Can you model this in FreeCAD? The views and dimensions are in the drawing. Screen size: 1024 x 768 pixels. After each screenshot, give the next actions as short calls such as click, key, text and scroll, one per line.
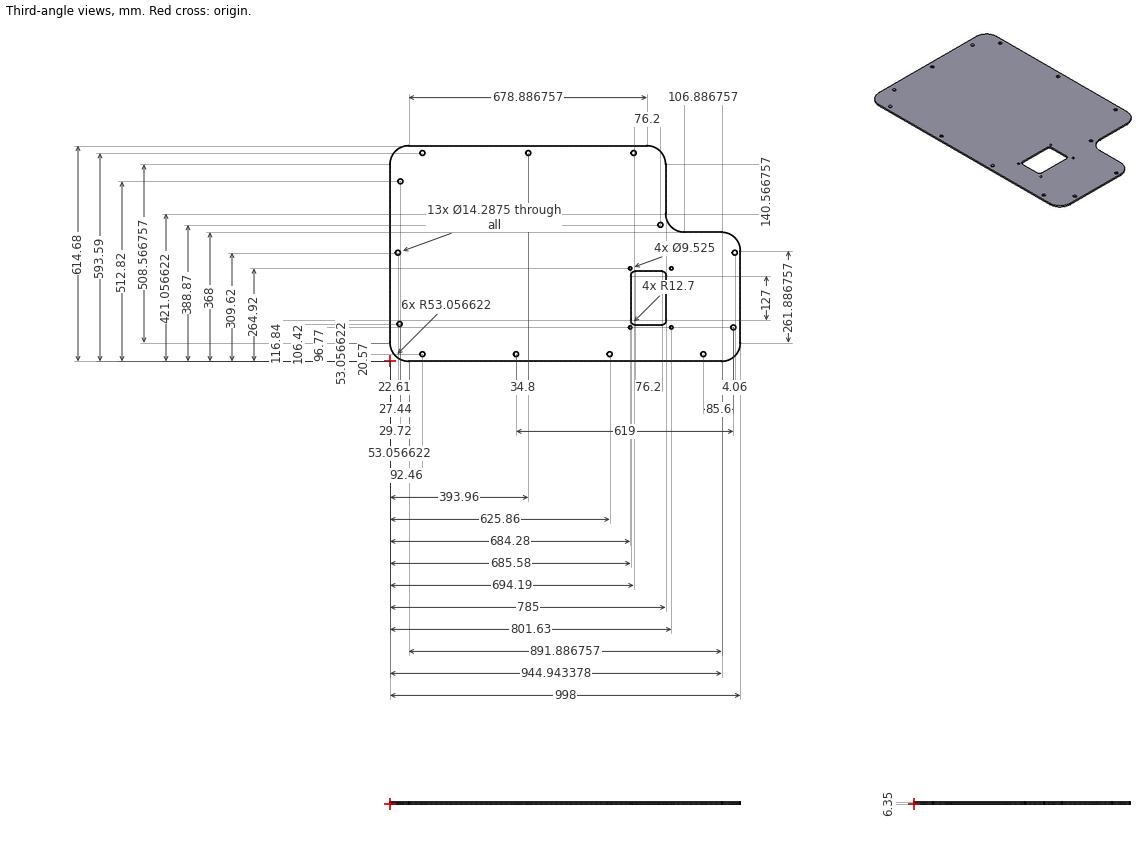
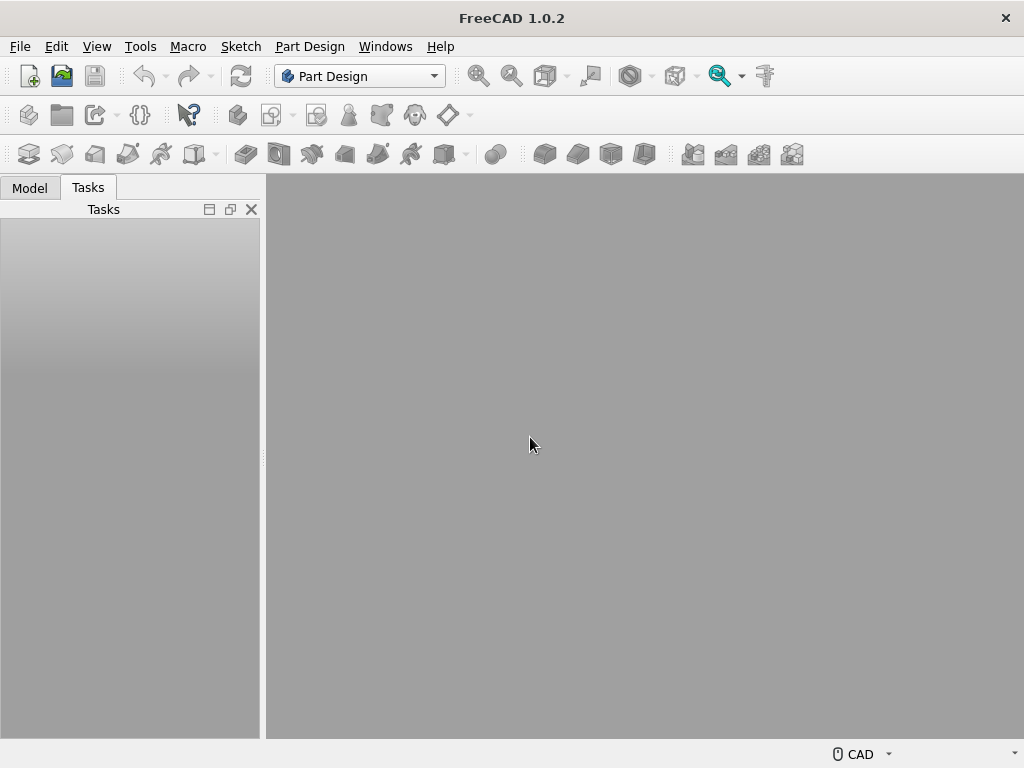
click(29, 76)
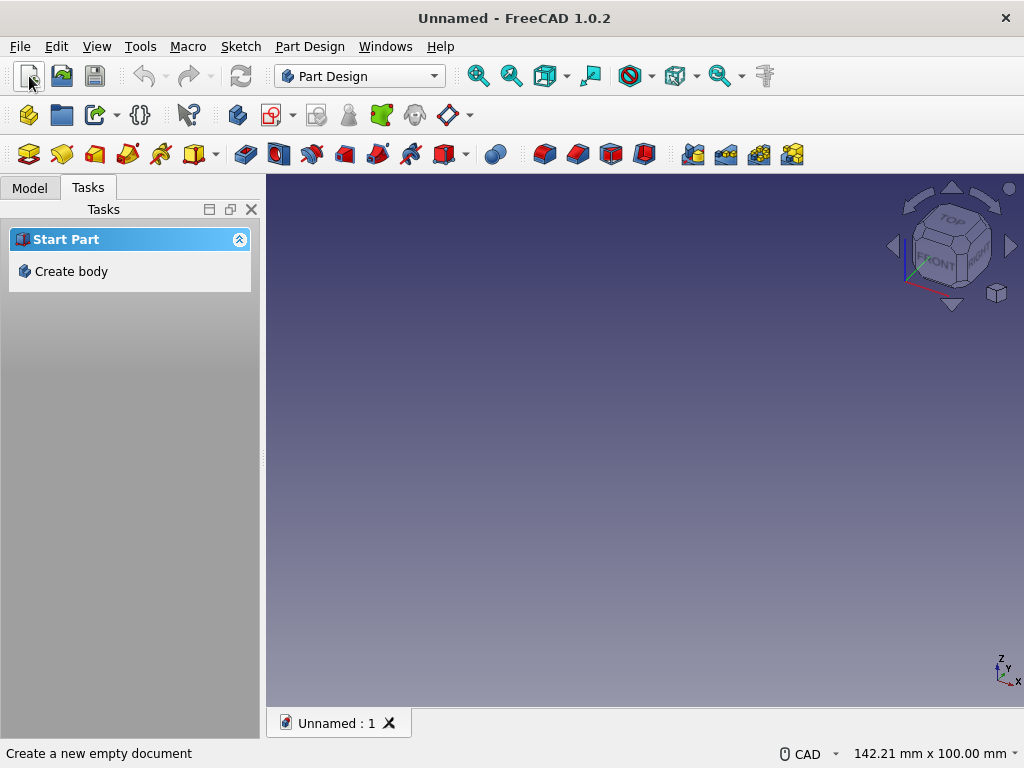
click(270, 116)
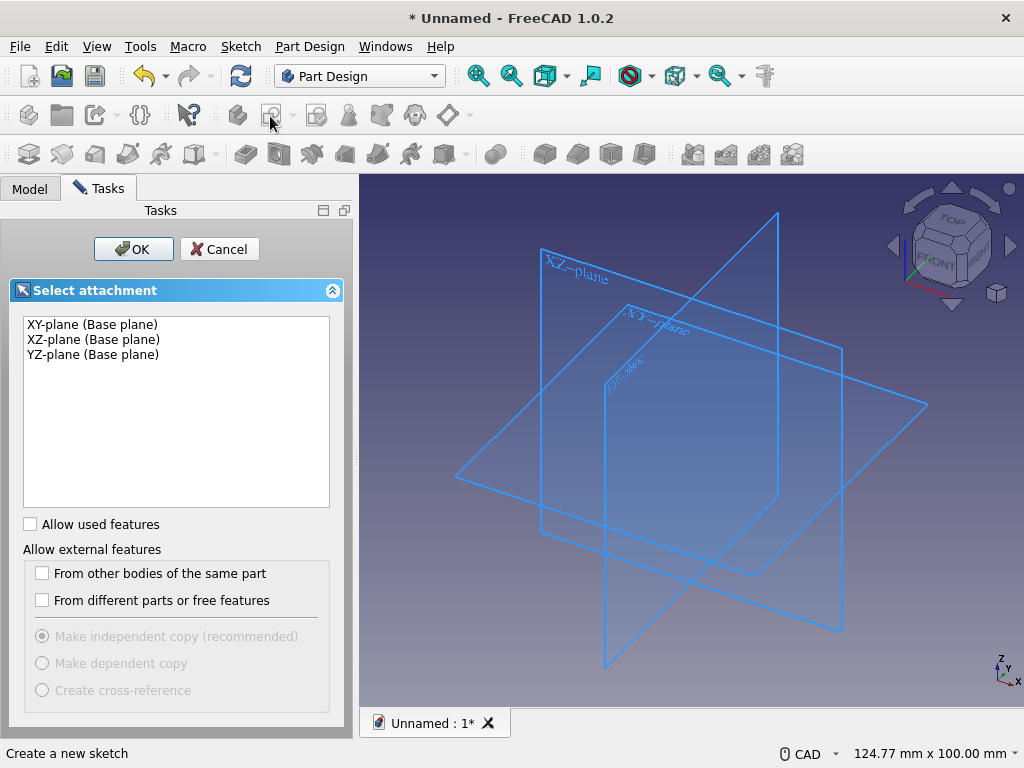
click(84, 324)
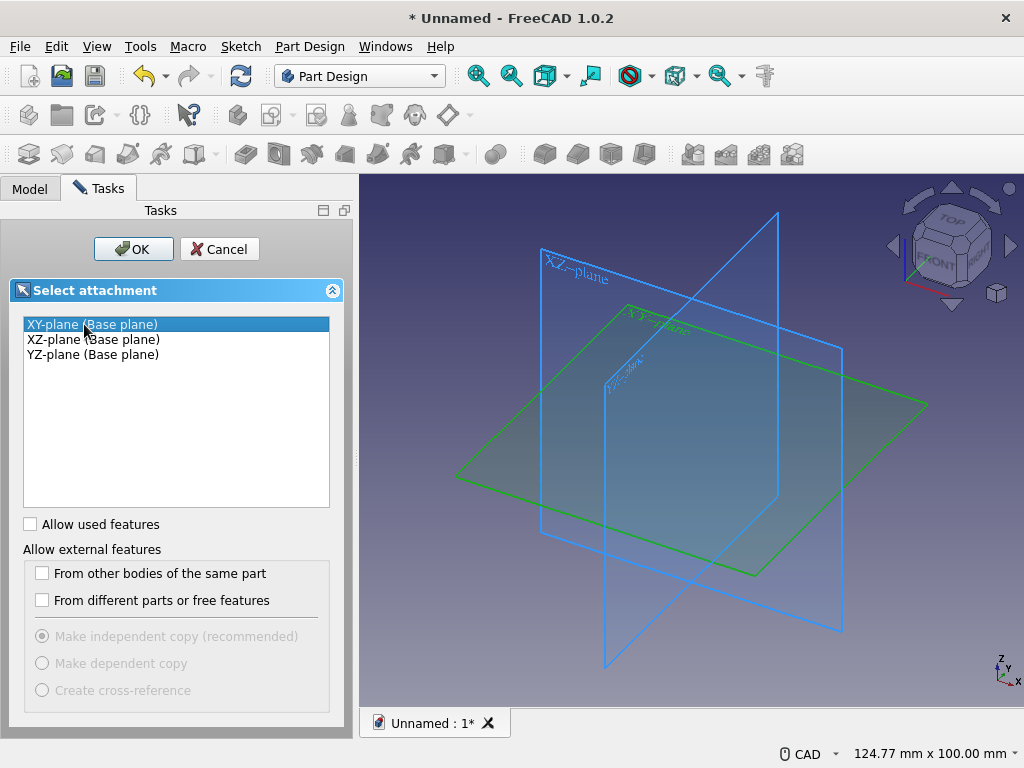
click(134, 249)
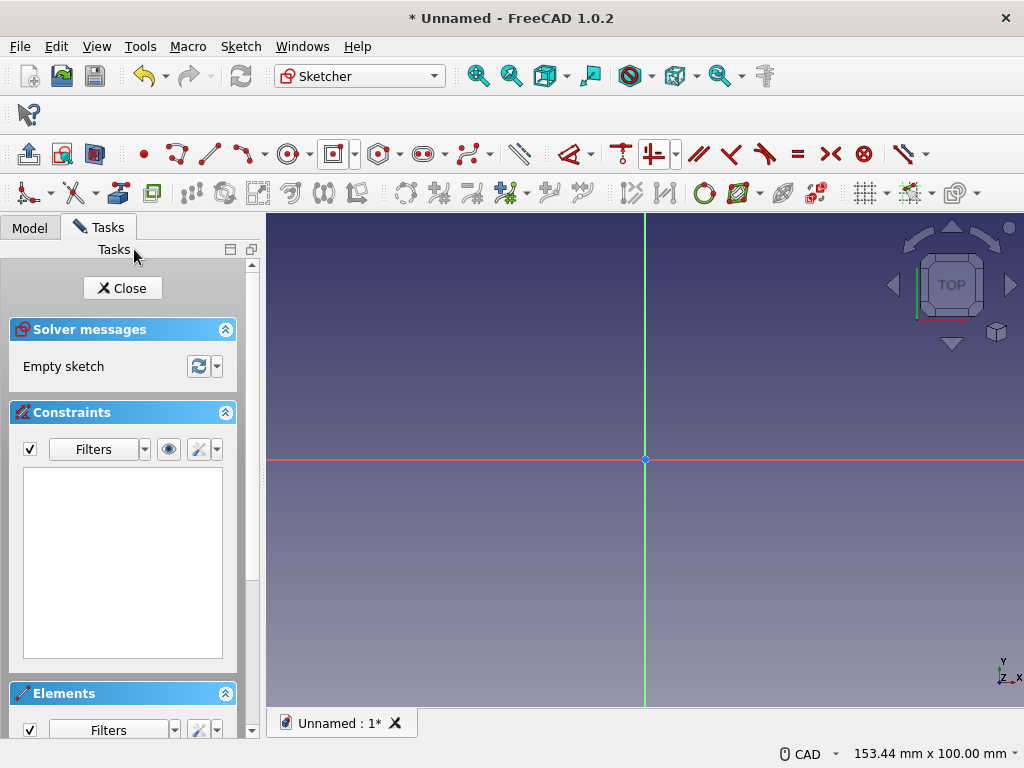
scroll(373, 582, down, 13)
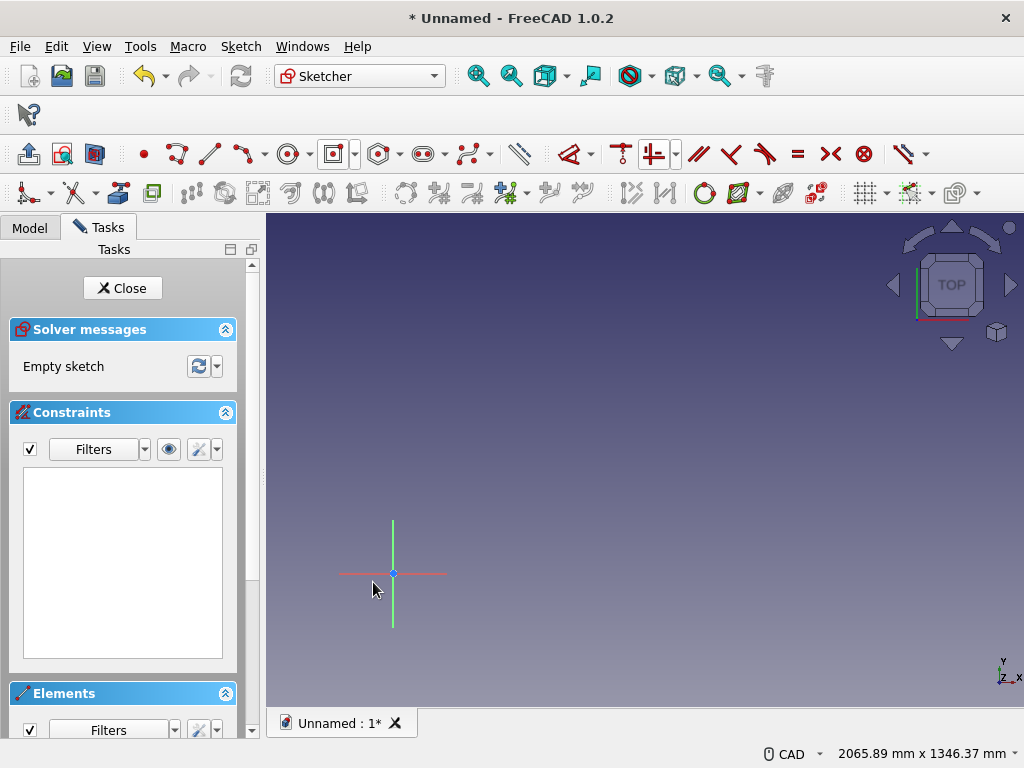
click(210, 154)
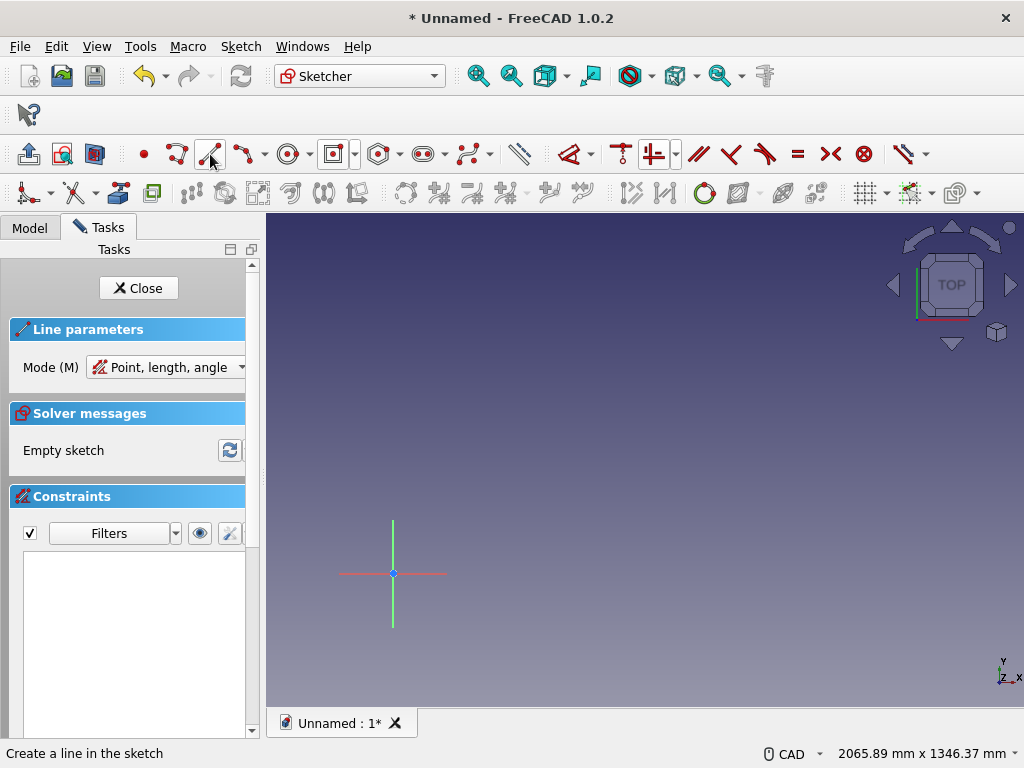
click(393, 368)
click(402, 554)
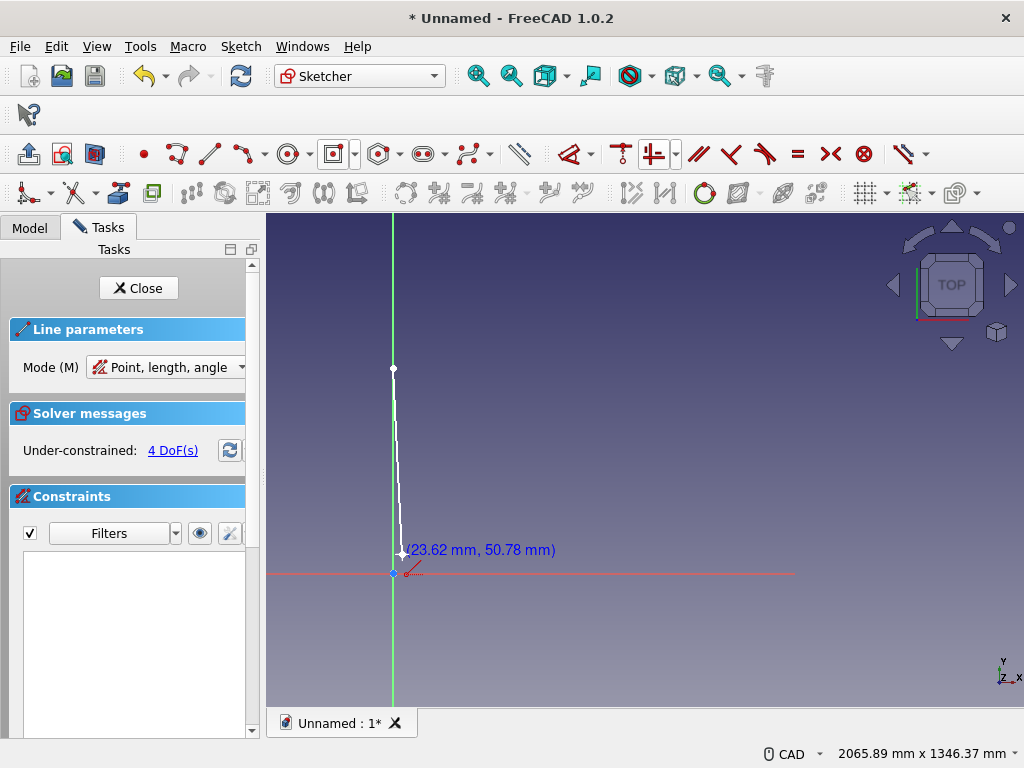
click(413, 574)
click(740, 565)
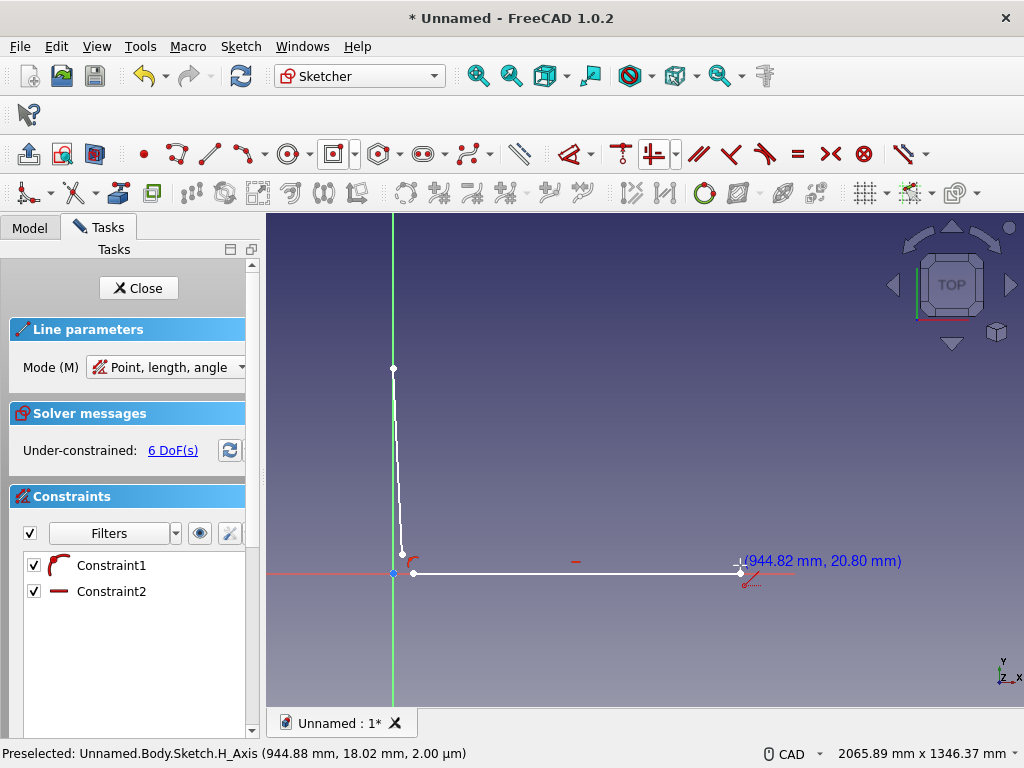
click(760, 554)
click(760, 458)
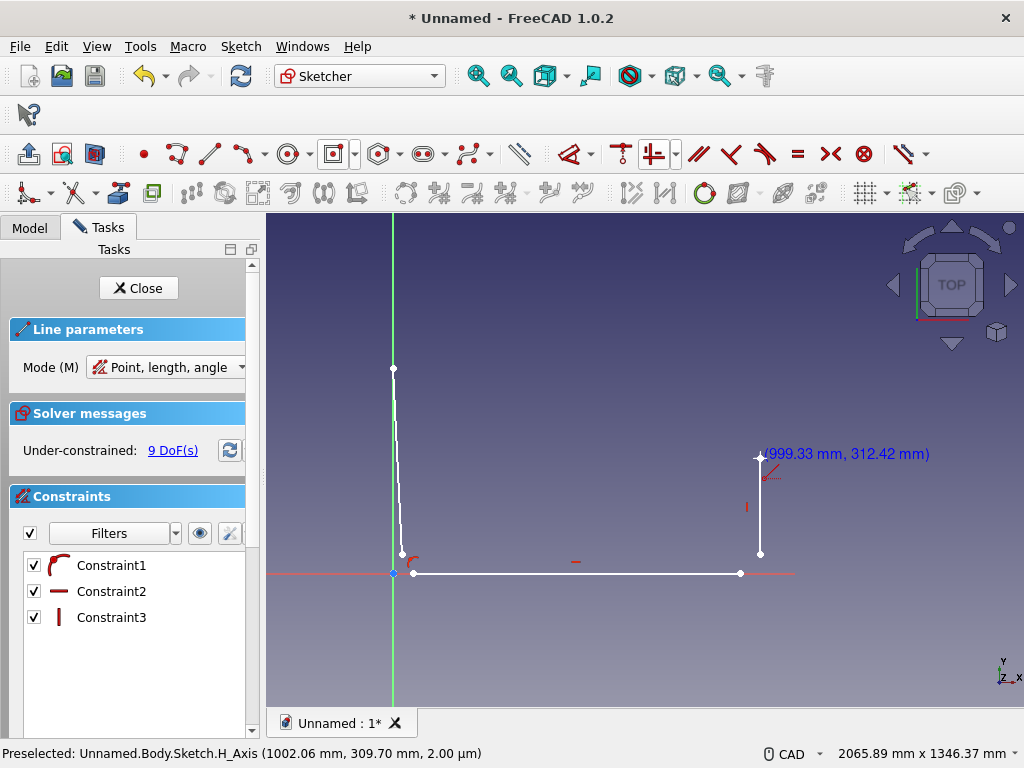
click(740, 439)
click(701, 439)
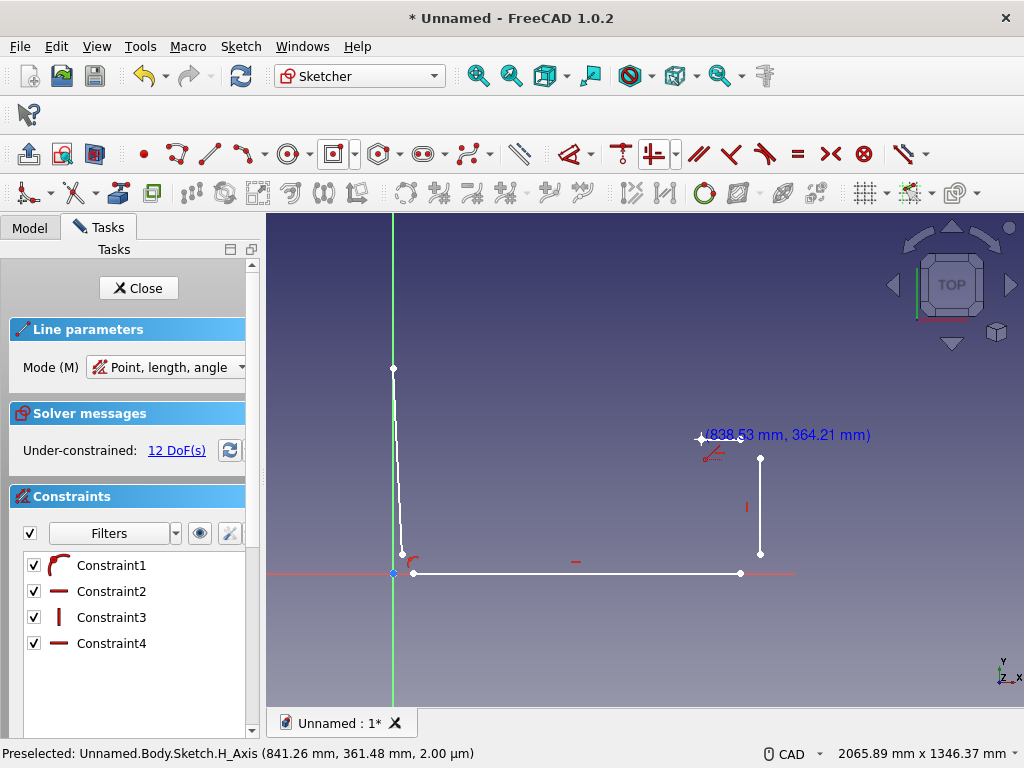
click(681, 419)
click(681, 368)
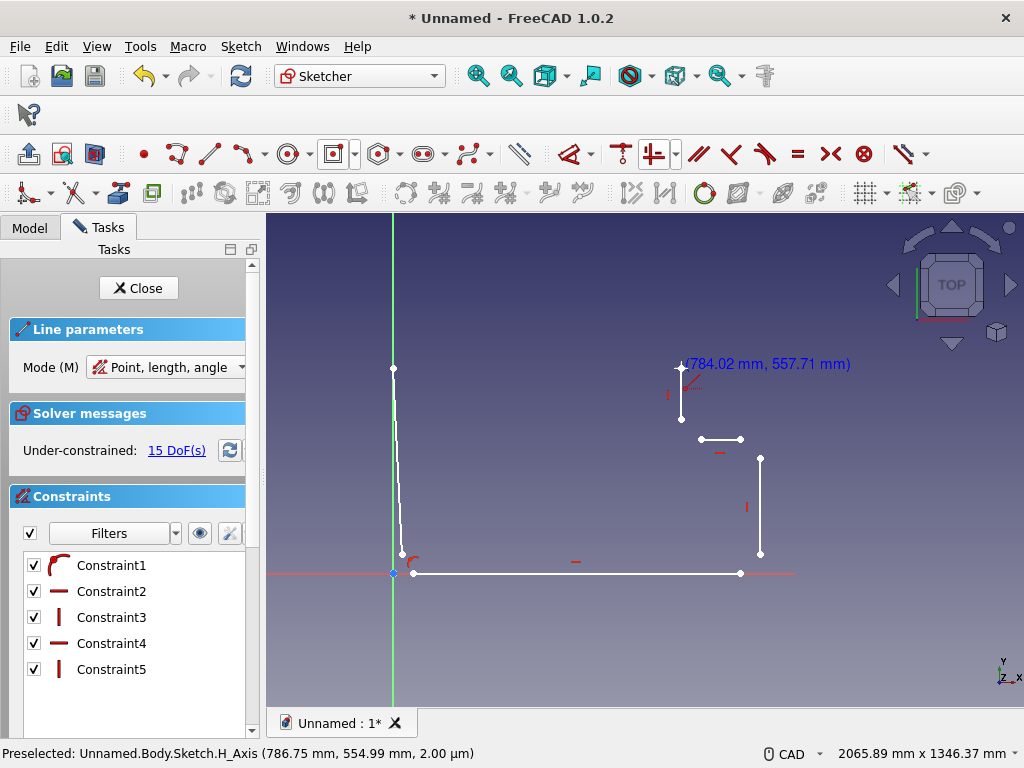
click(662, 348)
click(413, 348)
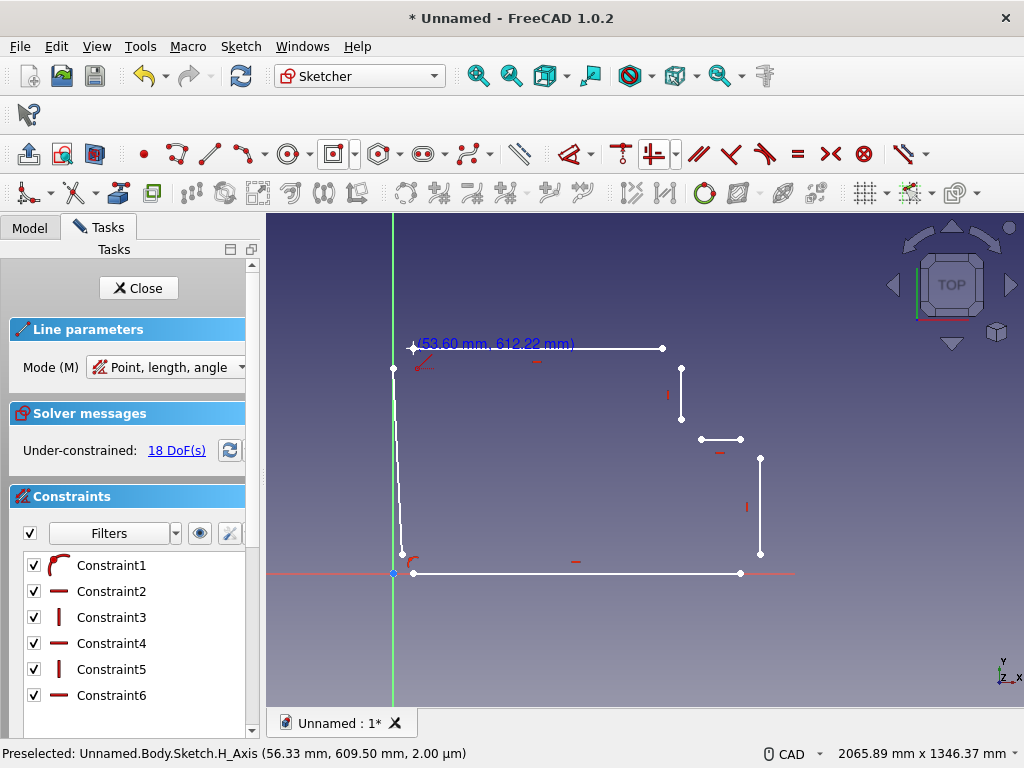
click(242, 154)